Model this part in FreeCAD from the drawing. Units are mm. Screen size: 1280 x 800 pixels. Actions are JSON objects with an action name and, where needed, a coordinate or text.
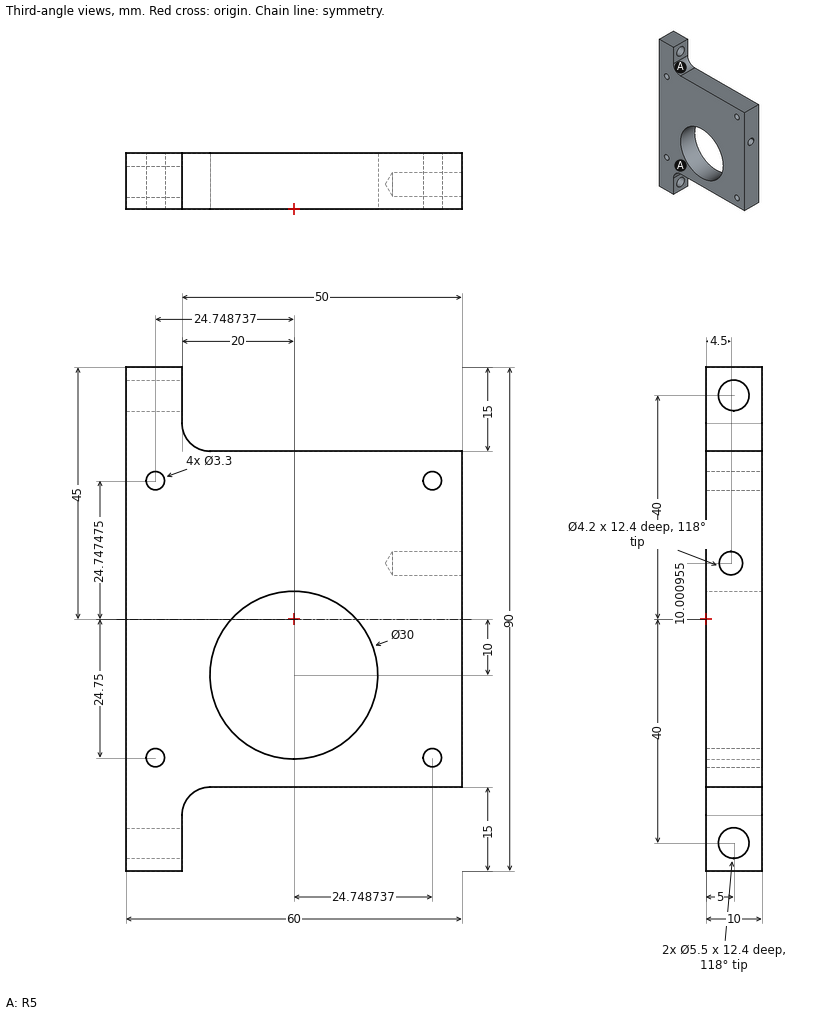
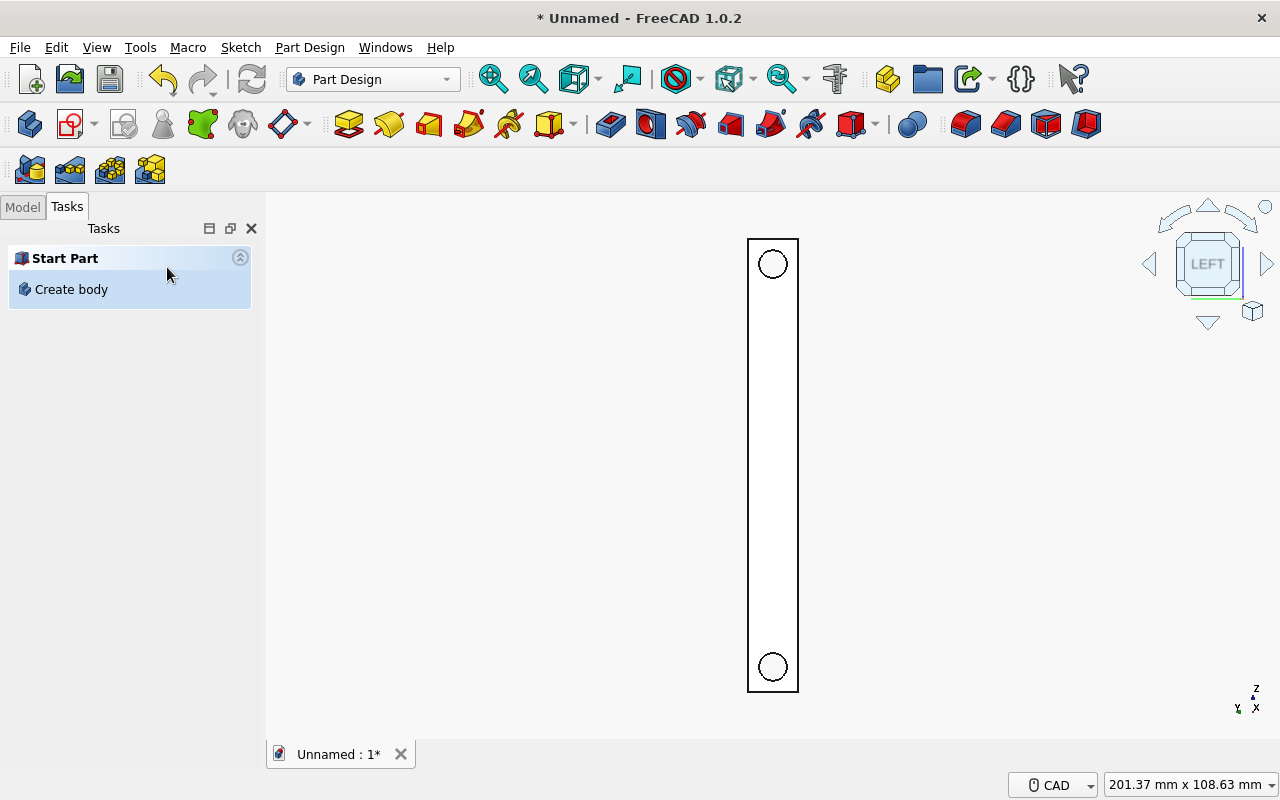
{"action": "key", "text": "v 3"}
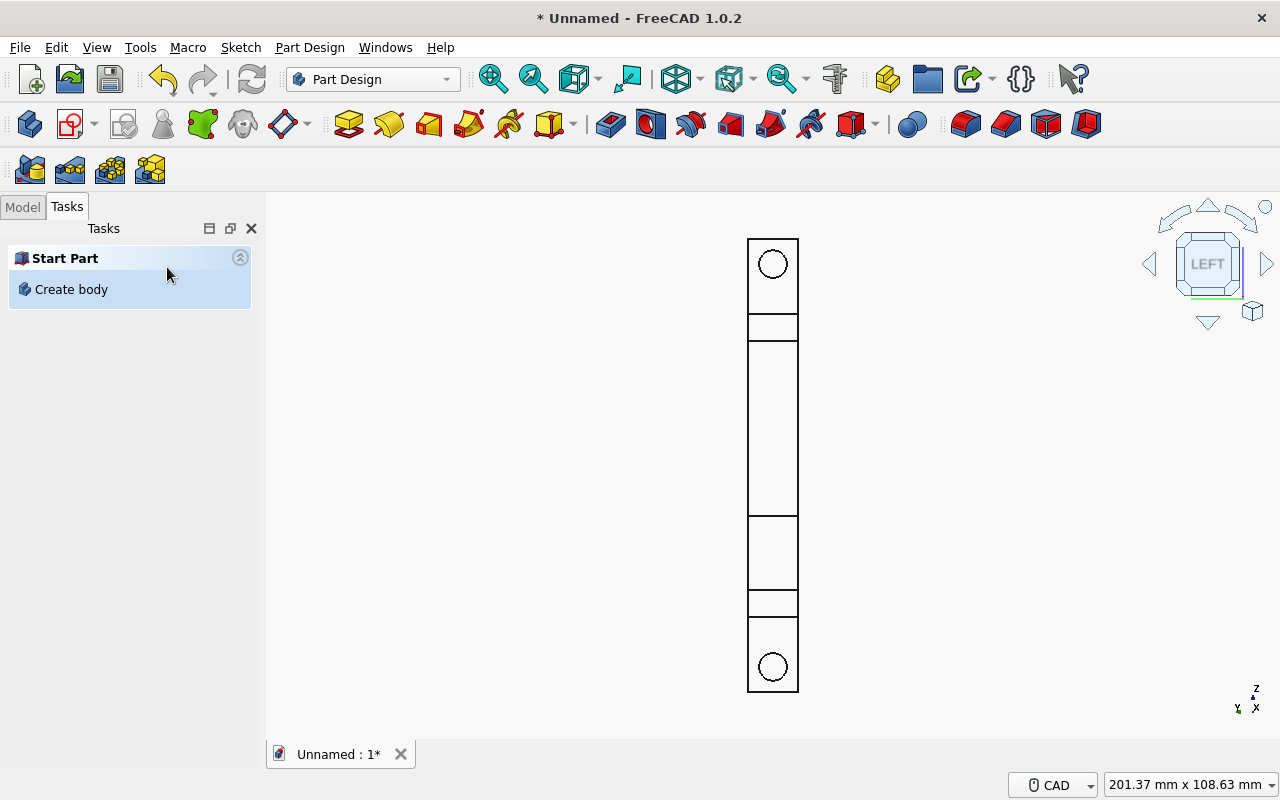
{"action": "key", "text": "0"}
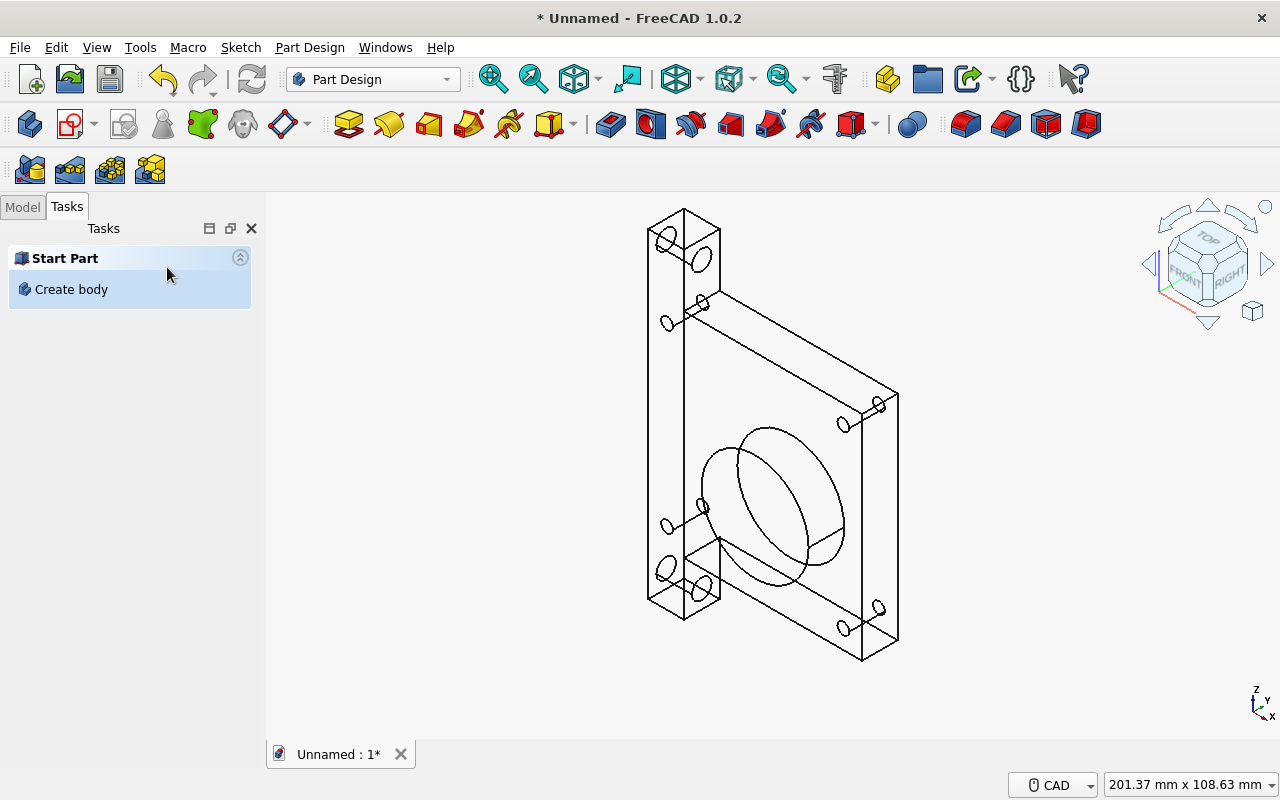
{"action": "left_click", "coordinate": [702, 300]}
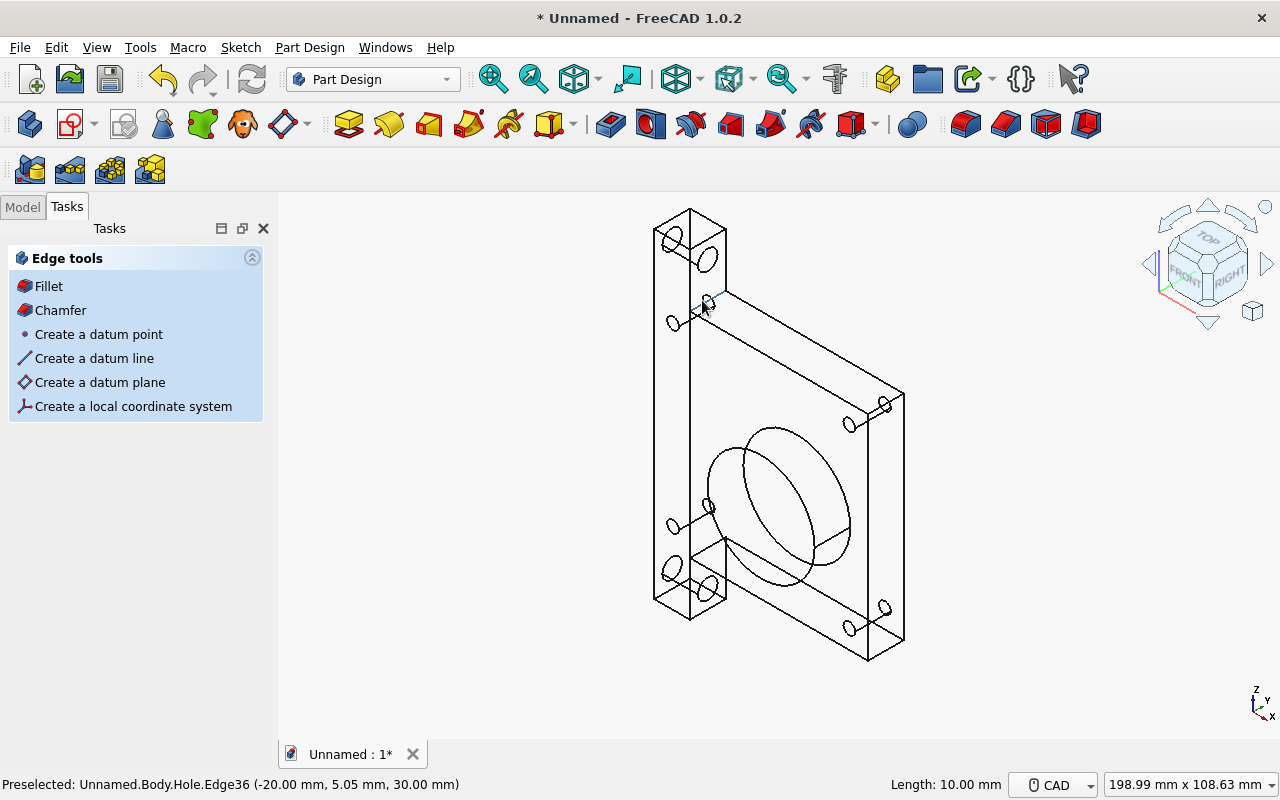
{"action": "left_click", "coordinate": [708, 547], "text": "ctrl"}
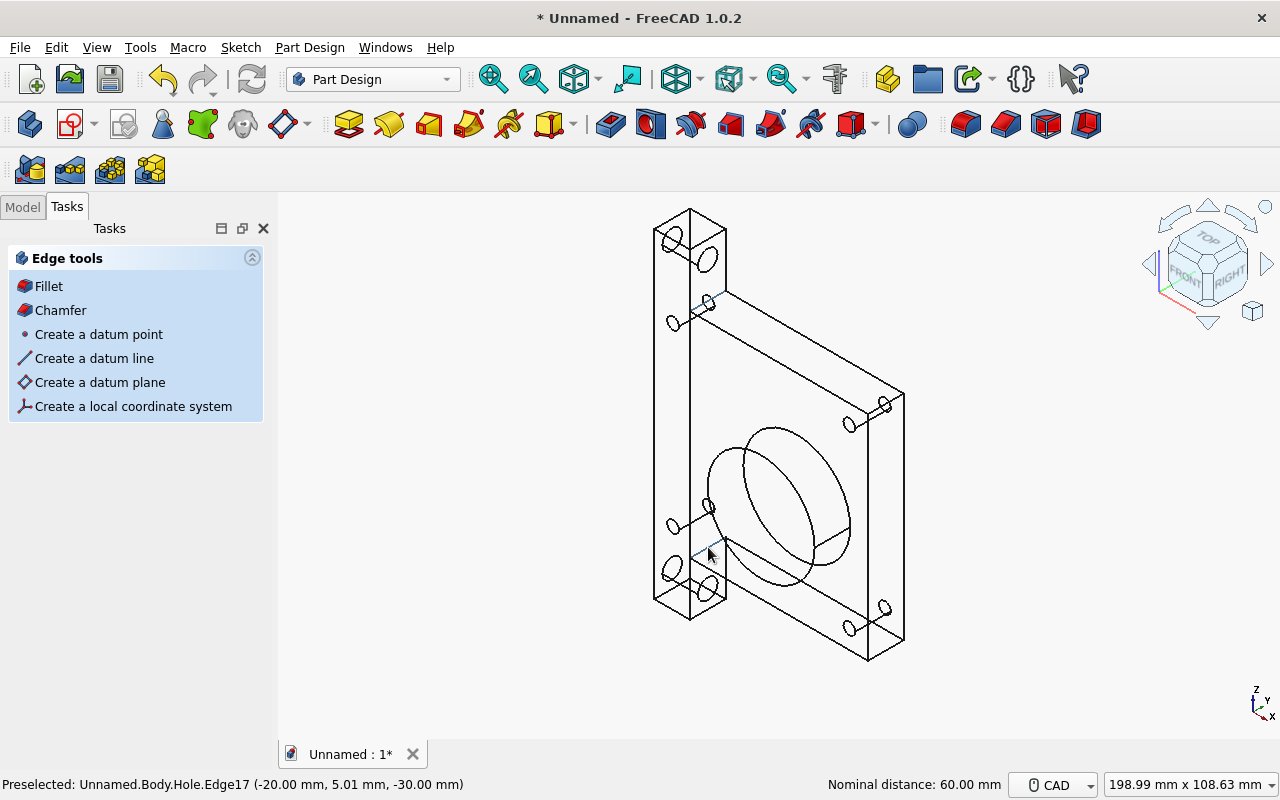
{"action": "key", "text": "v 1"}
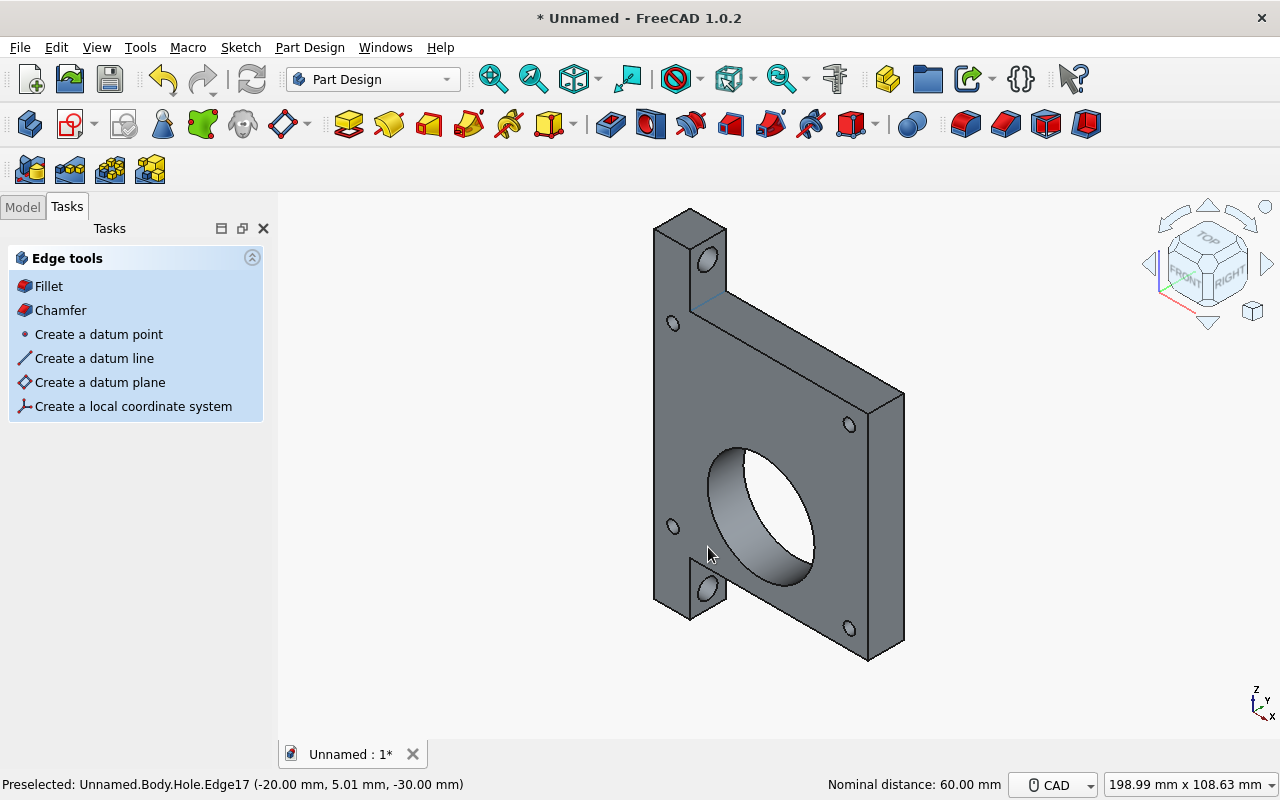
{"action": "left_click", "coordinate": [966, 124]}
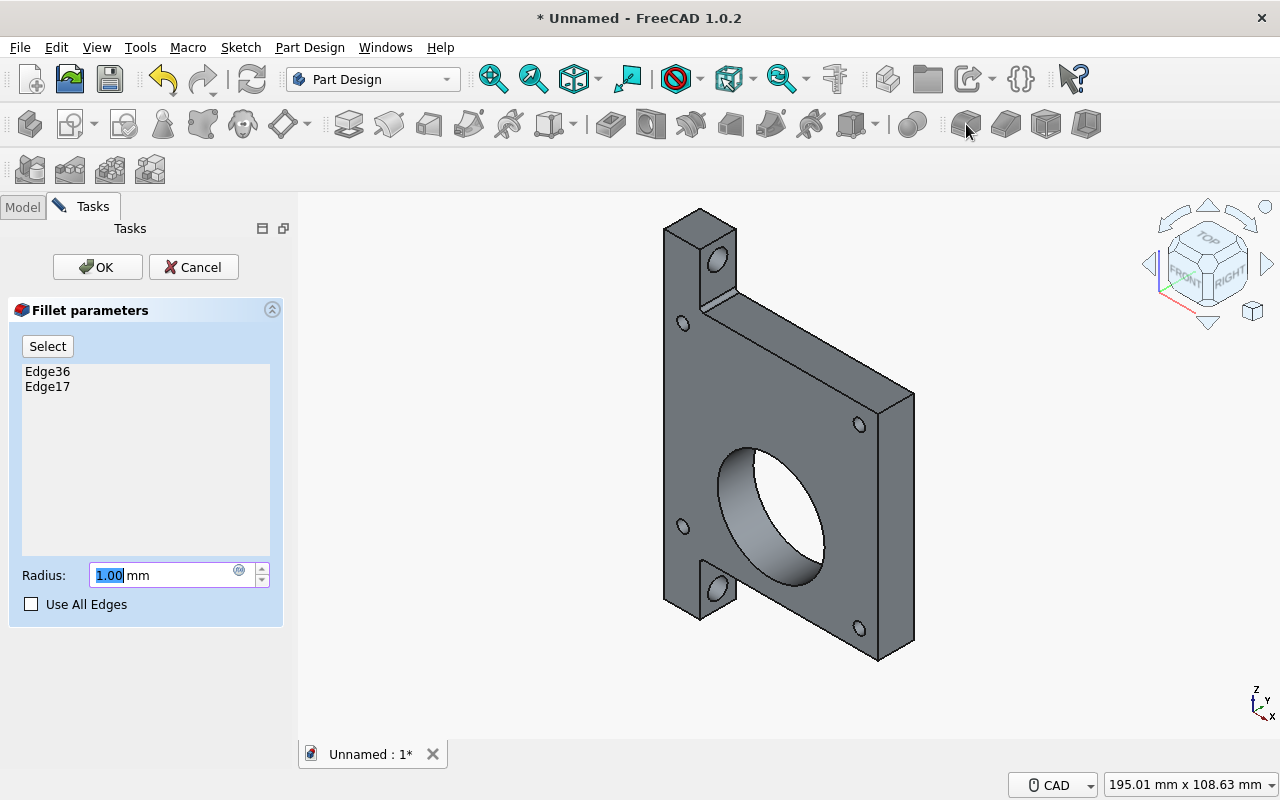
{"action": "type", "text": "5"}
{"action": "key", "text": "Tab"}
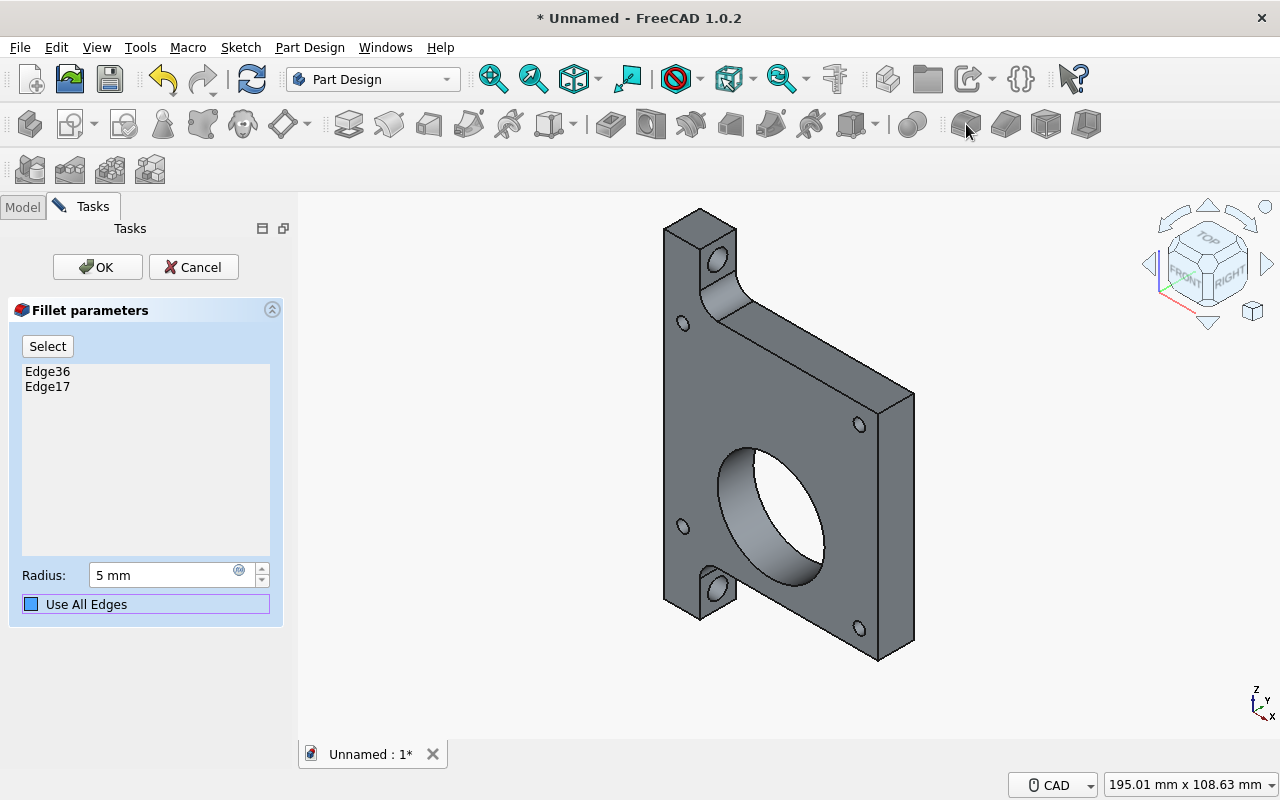
{"action": "left_click", "coordinate": [98, 267]}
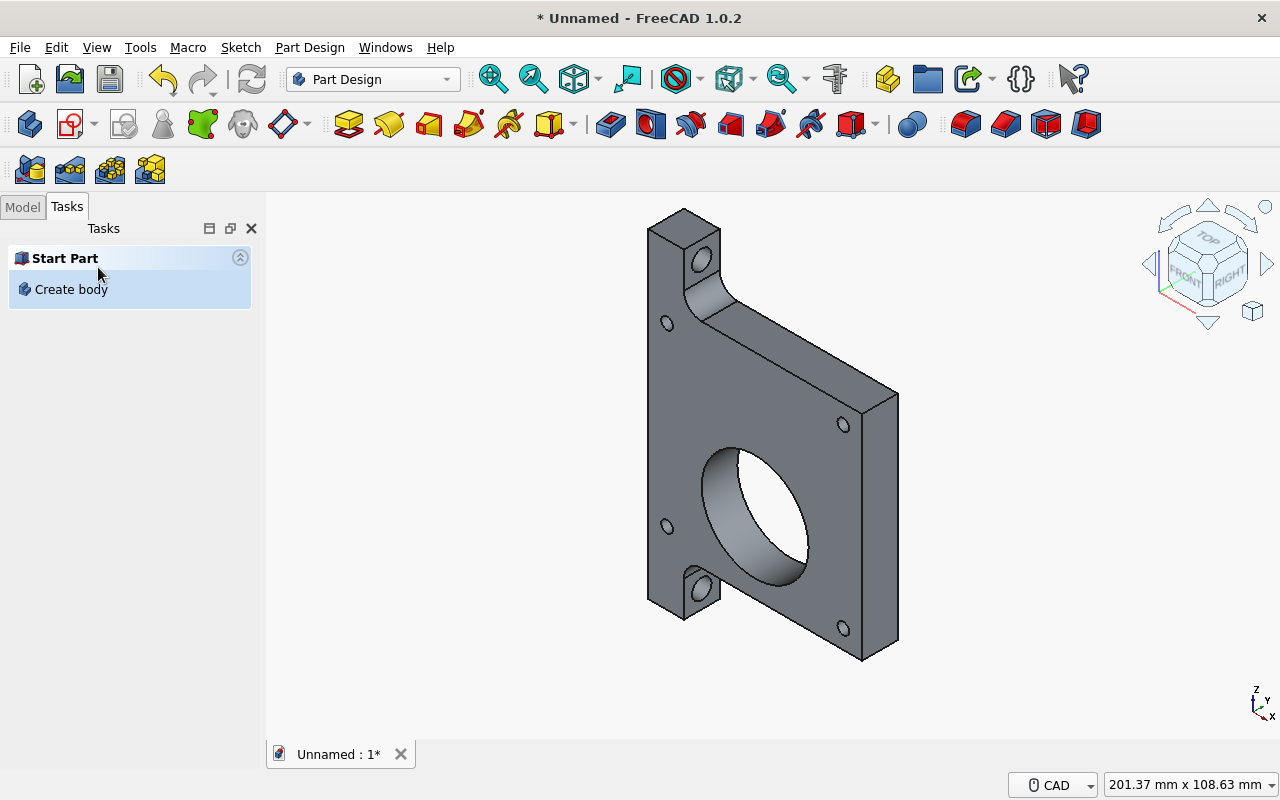
{"action": "left_click", "coordinate": [880, 561]}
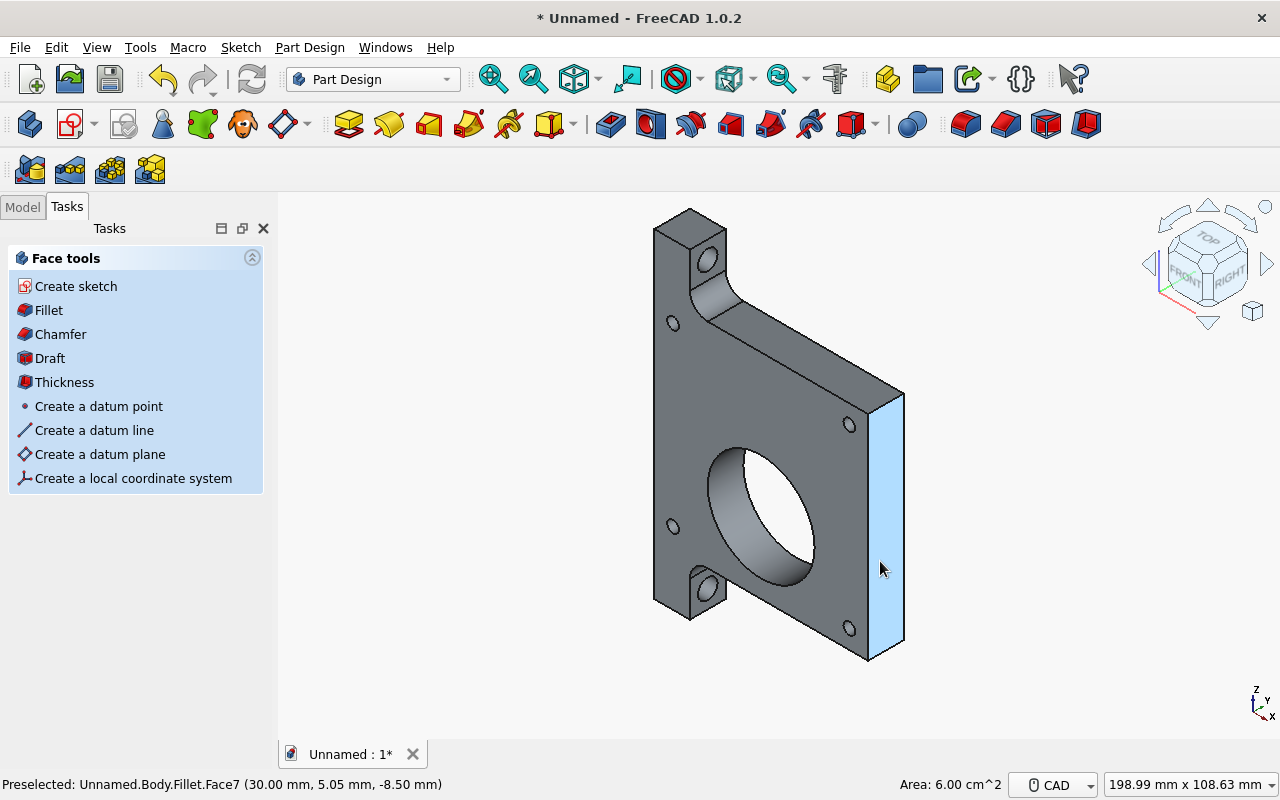
{"action": "left_click", "coordinate": [70, 124]}